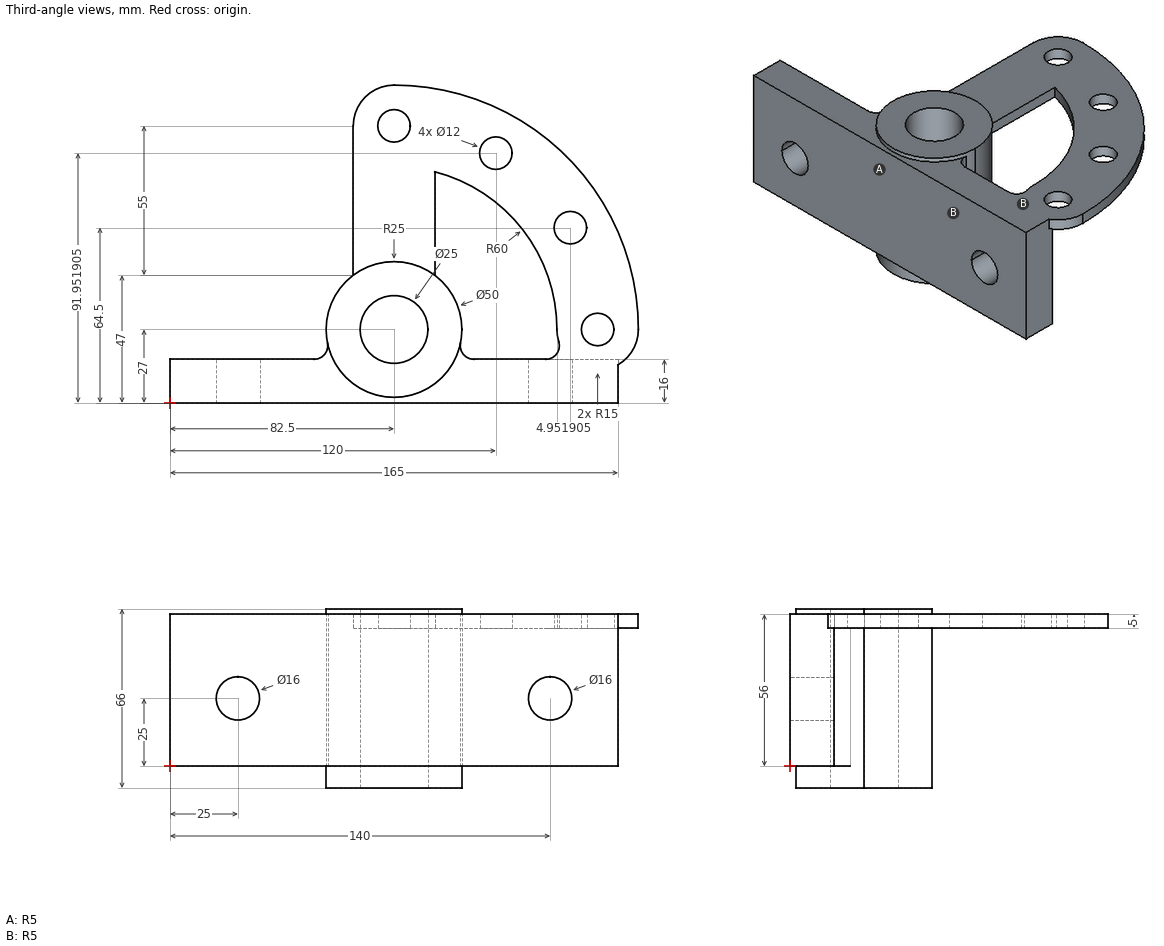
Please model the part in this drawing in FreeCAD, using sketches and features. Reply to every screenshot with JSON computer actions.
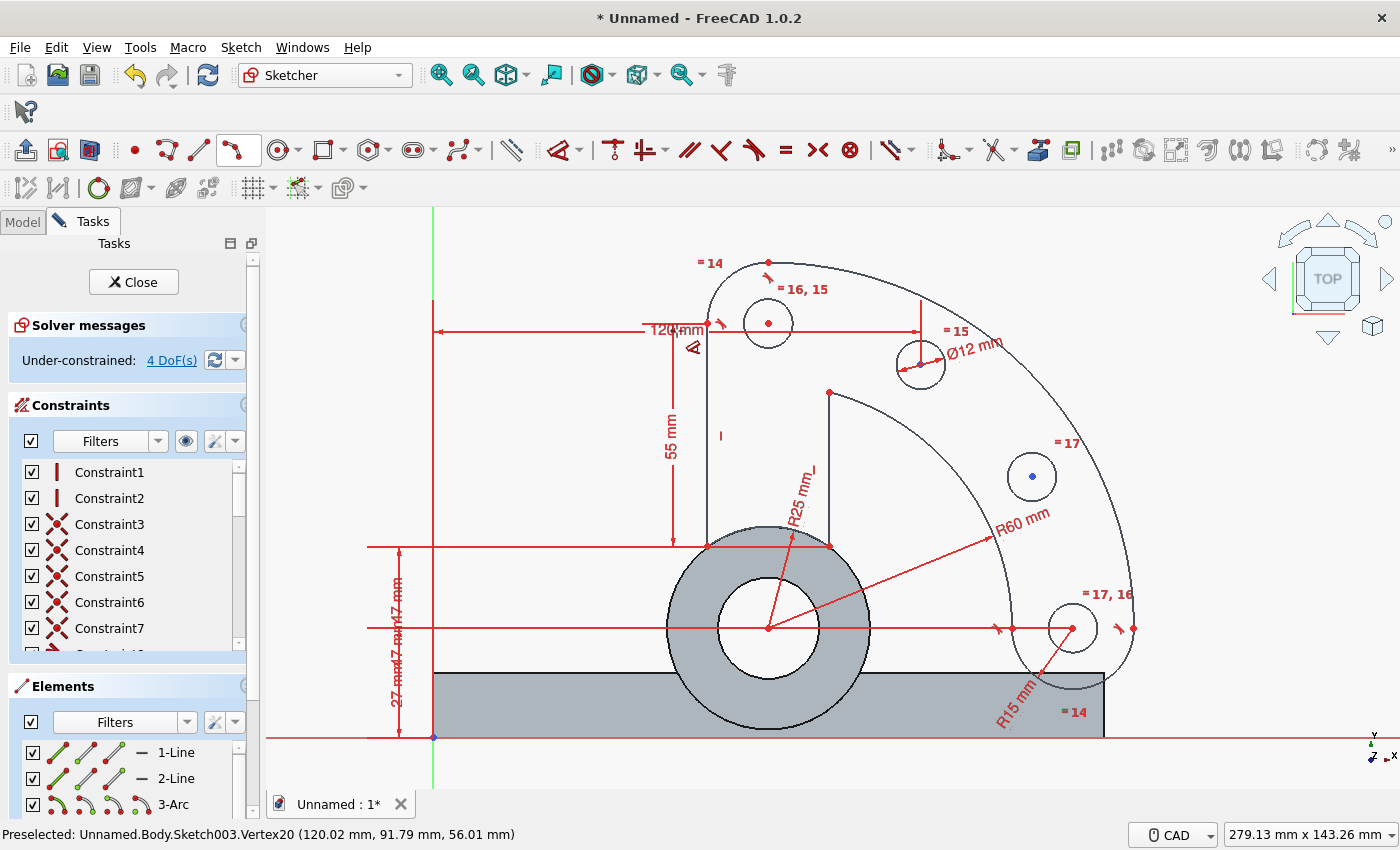
{"action": "left_click", "coordinate": [768, 324]}
{"action": "left_click", "coordinate": [601, 290]}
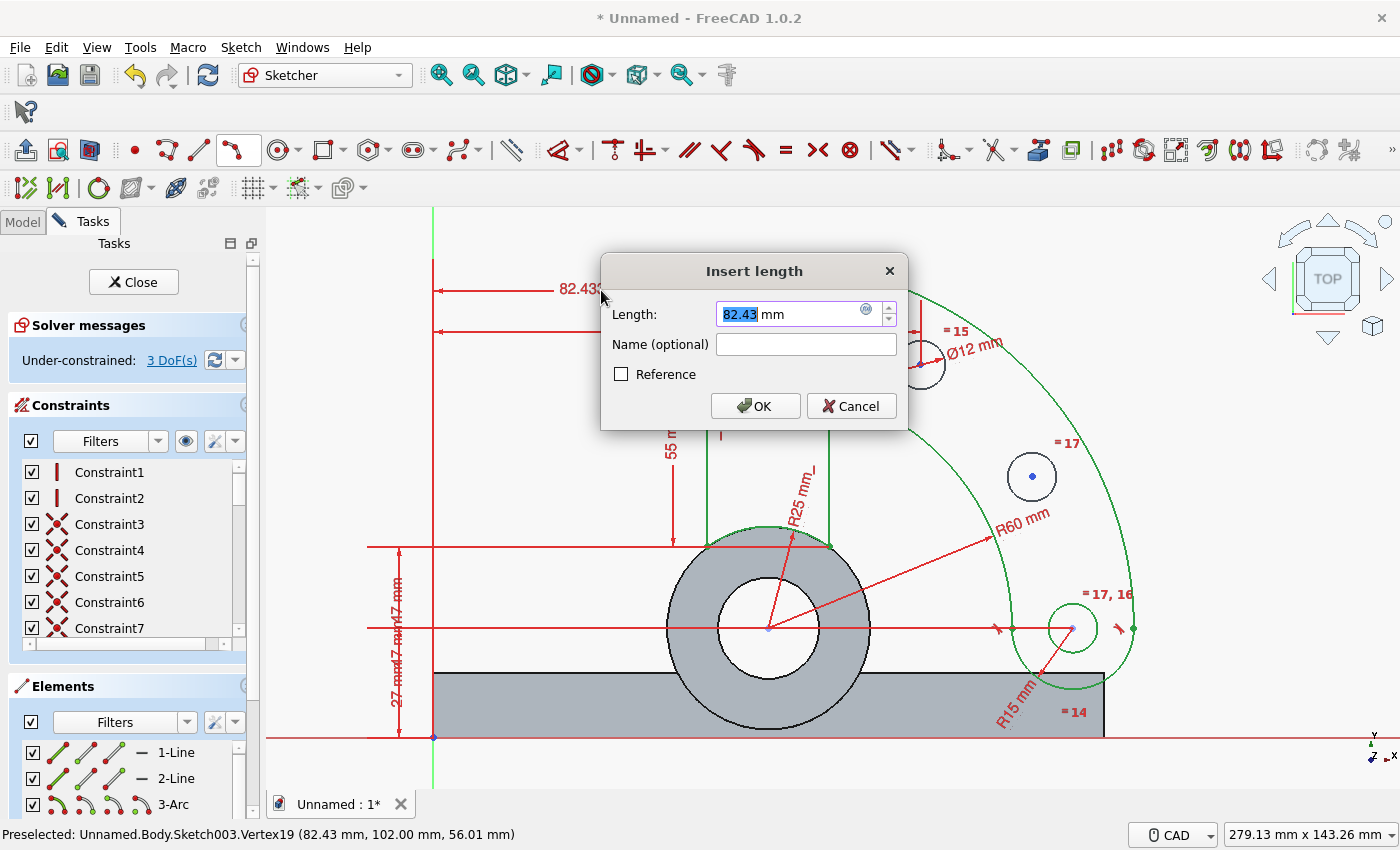
{"action": "type", "text": "82.5"}
{"action": "key", "text": "Return"}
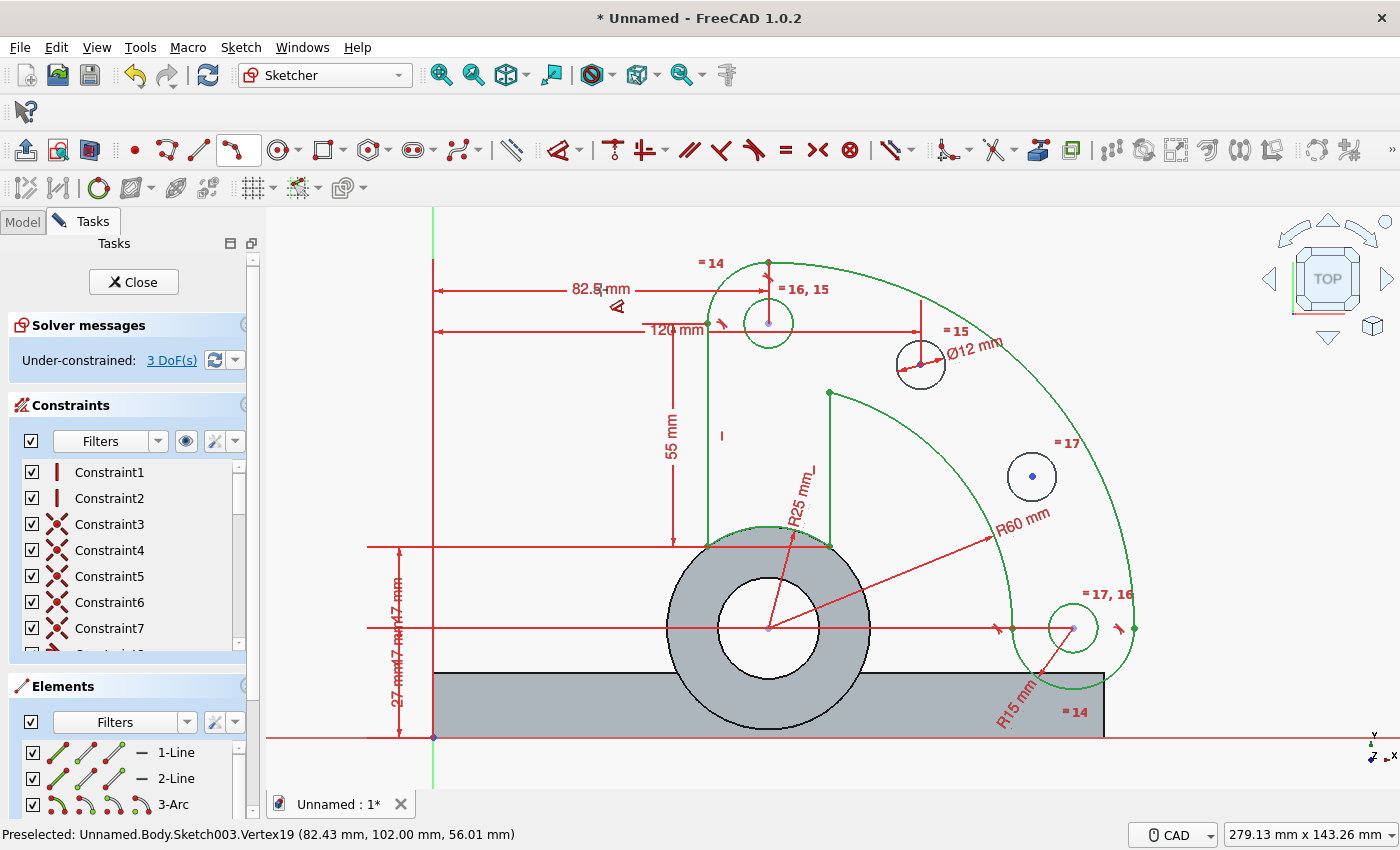
{"action": "left_click", "coordinate": [1032, 477]}
{"action": "left_click", "coordinate": [399, 547]}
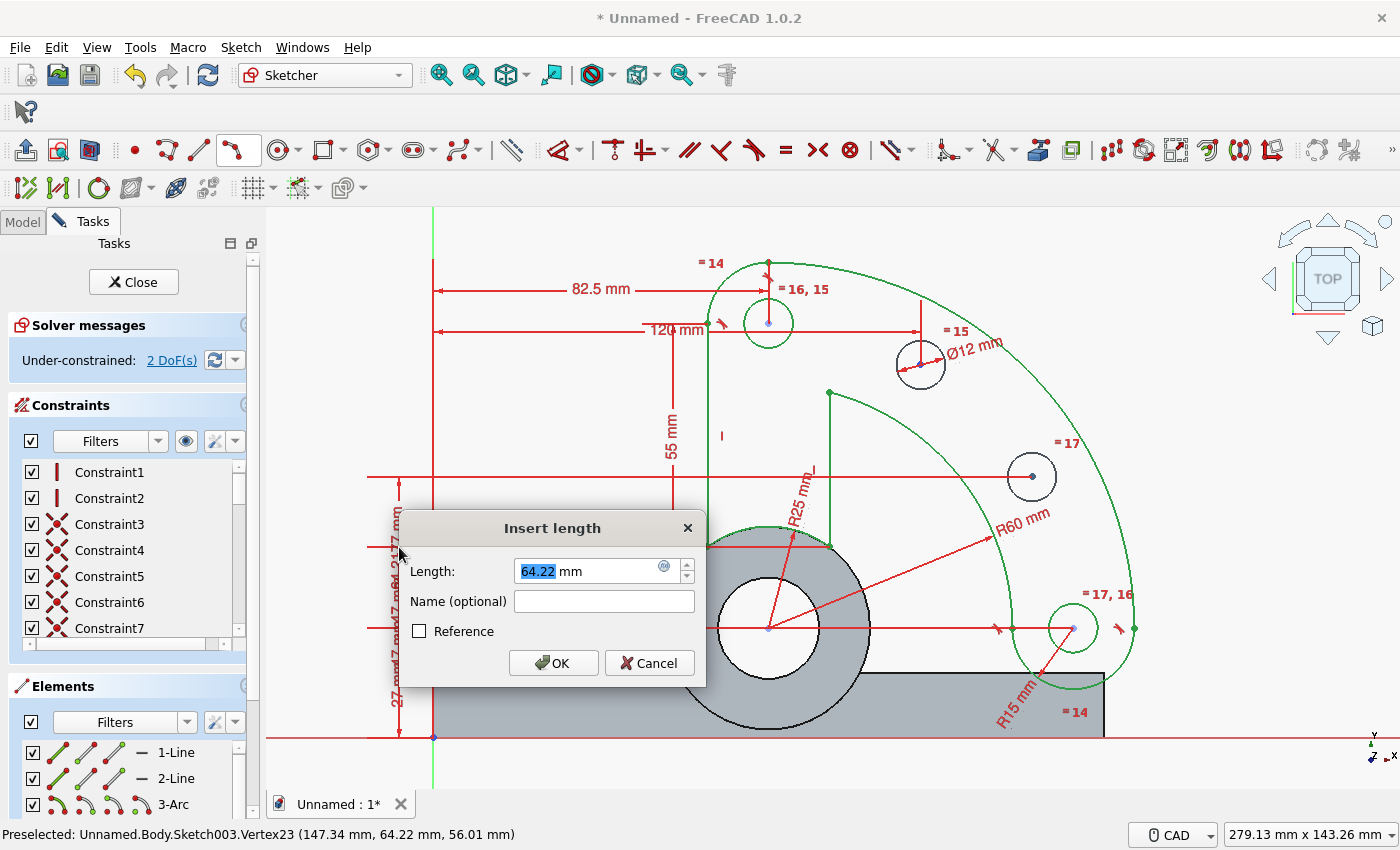
{"action": "type", "text": "64.5"}
{"action": "key", "text": "Return"}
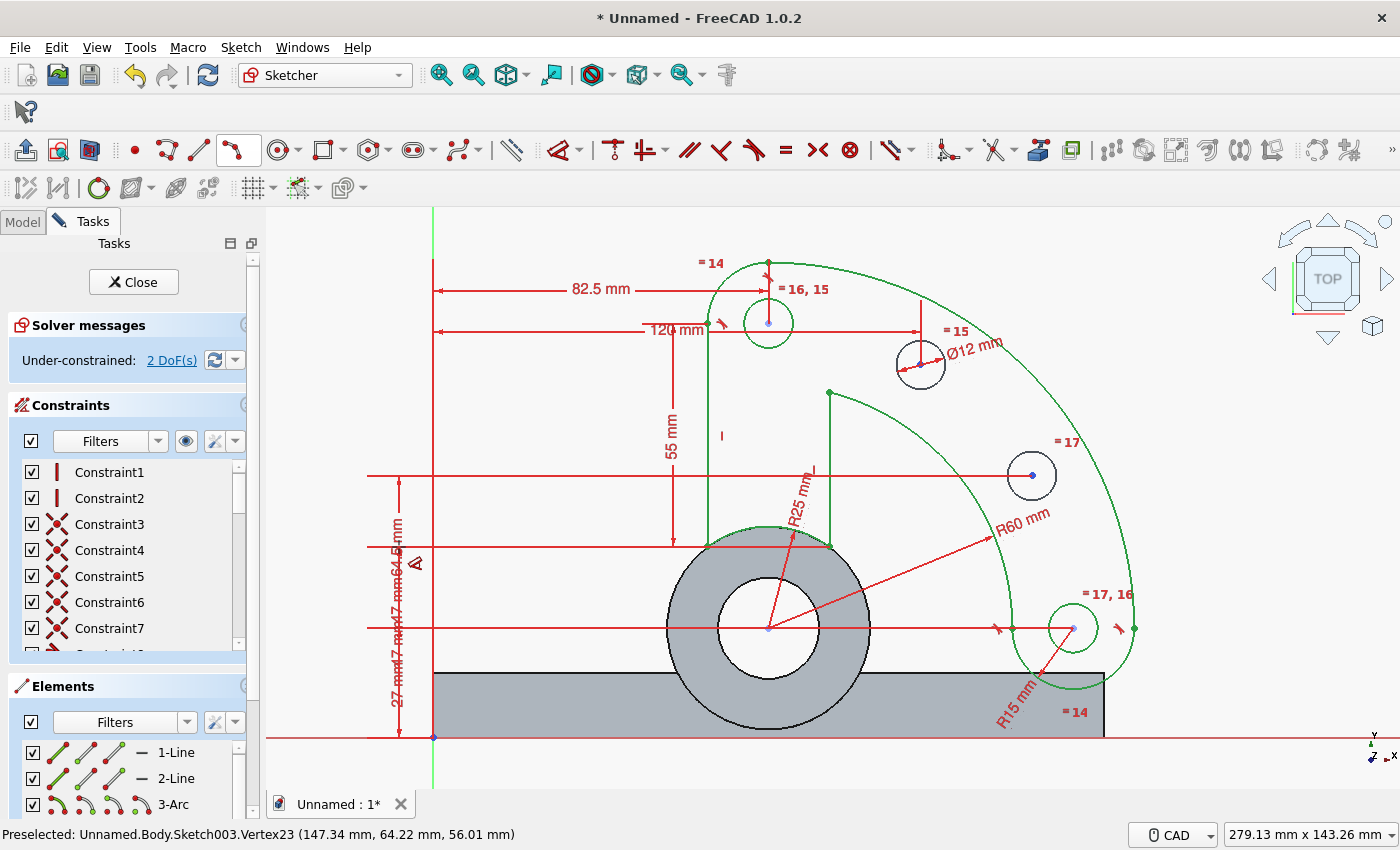
{"action": "left_click", "coordinate": [921, 365]}
{"action": "left_click", "coordinate": [399, 466]}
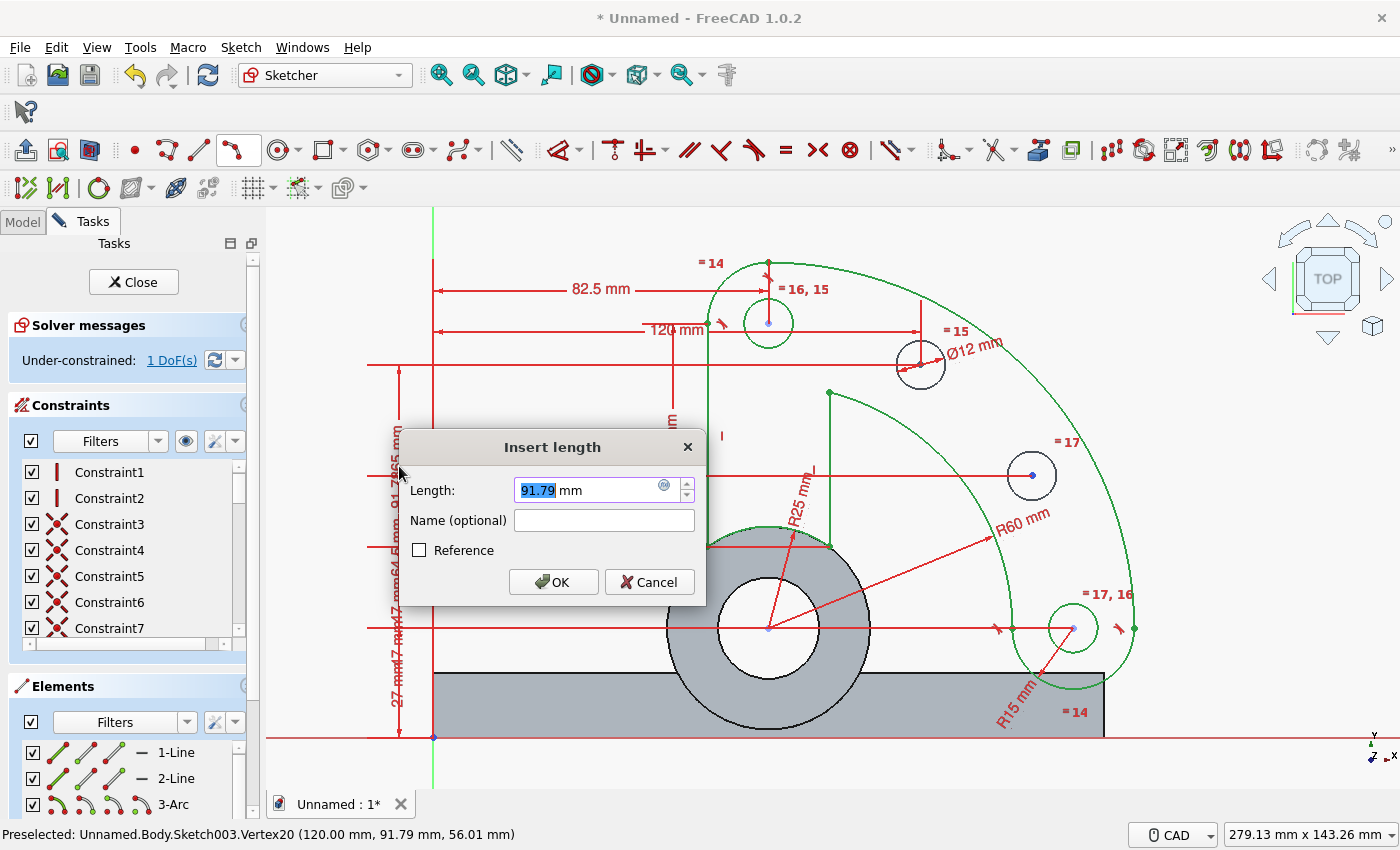
{"action": "type", "text": "91.951905"}
{"action": "key", "text": "Return"}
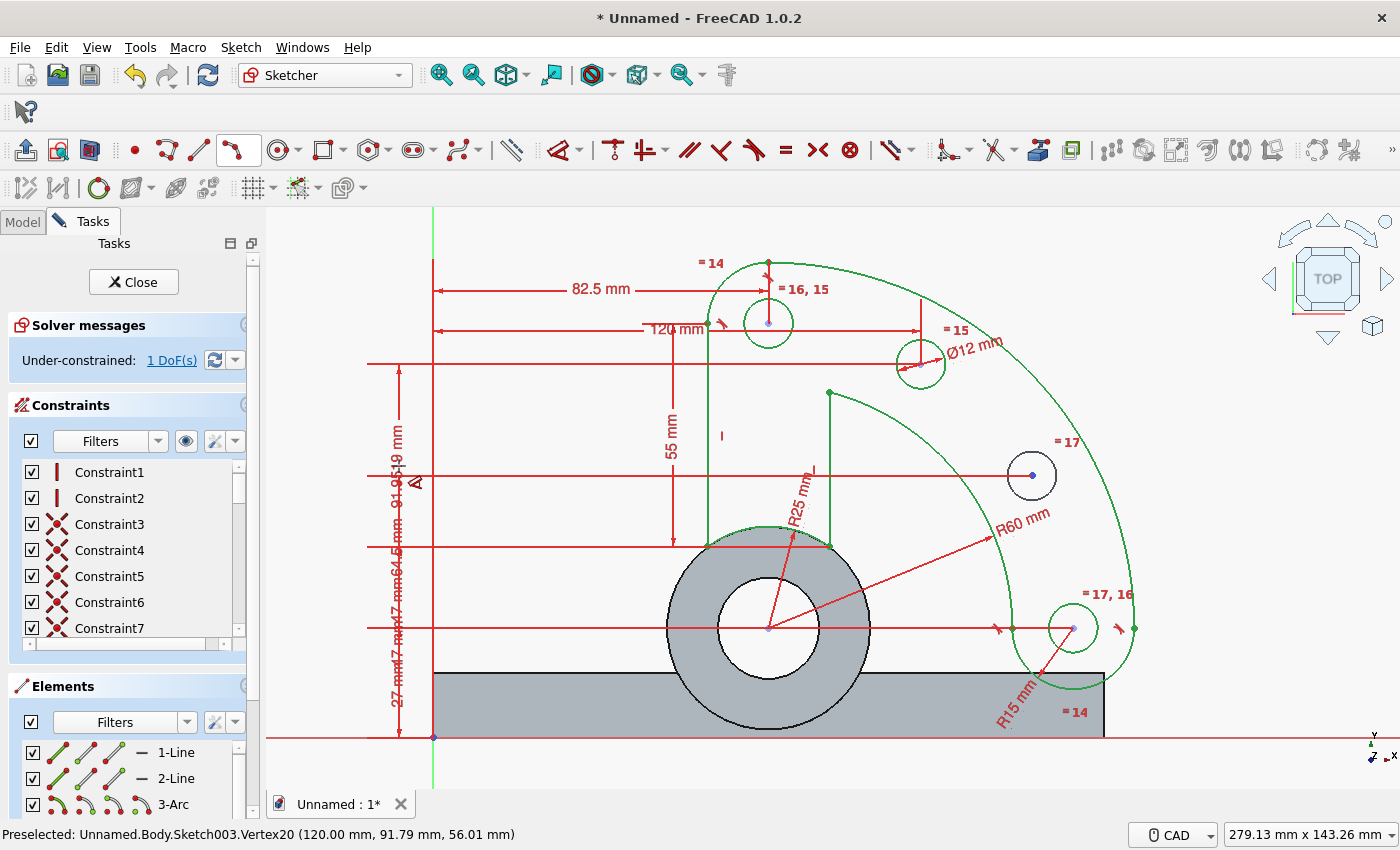
{"action": "scroll", "coordinate": [1012, 628], "scroll_direction": "up", "scroll_amount": 4}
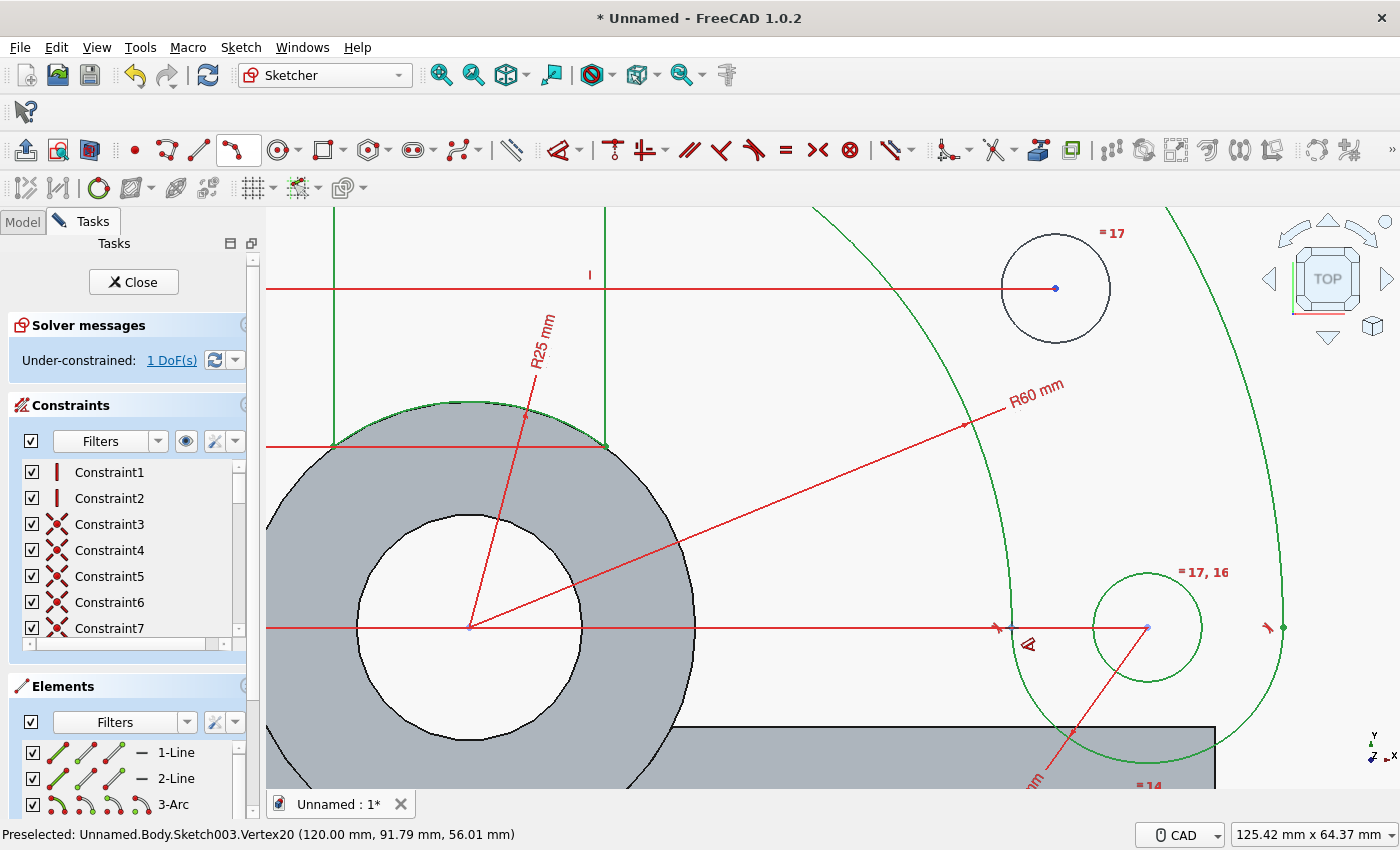
{"action": "left_click", "coordinate": [1012, 628]}